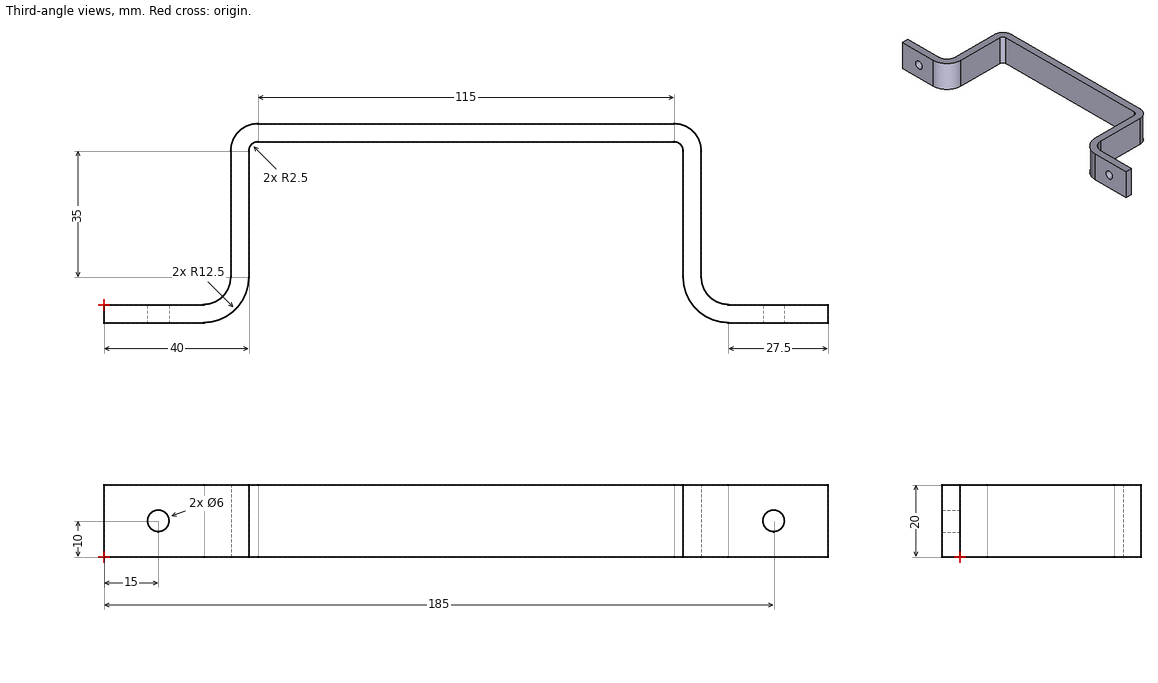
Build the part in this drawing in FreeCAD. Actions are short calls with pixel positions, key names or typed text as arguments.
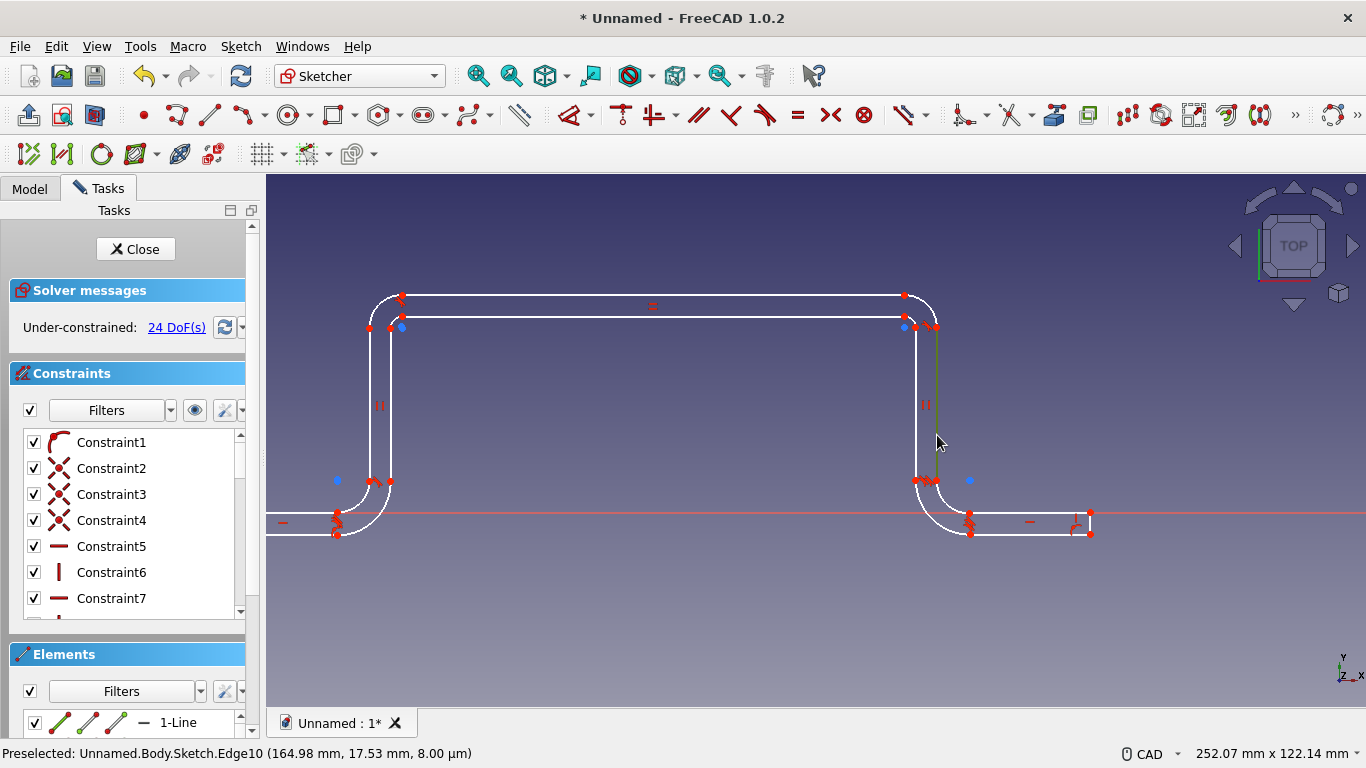
click(933, 313)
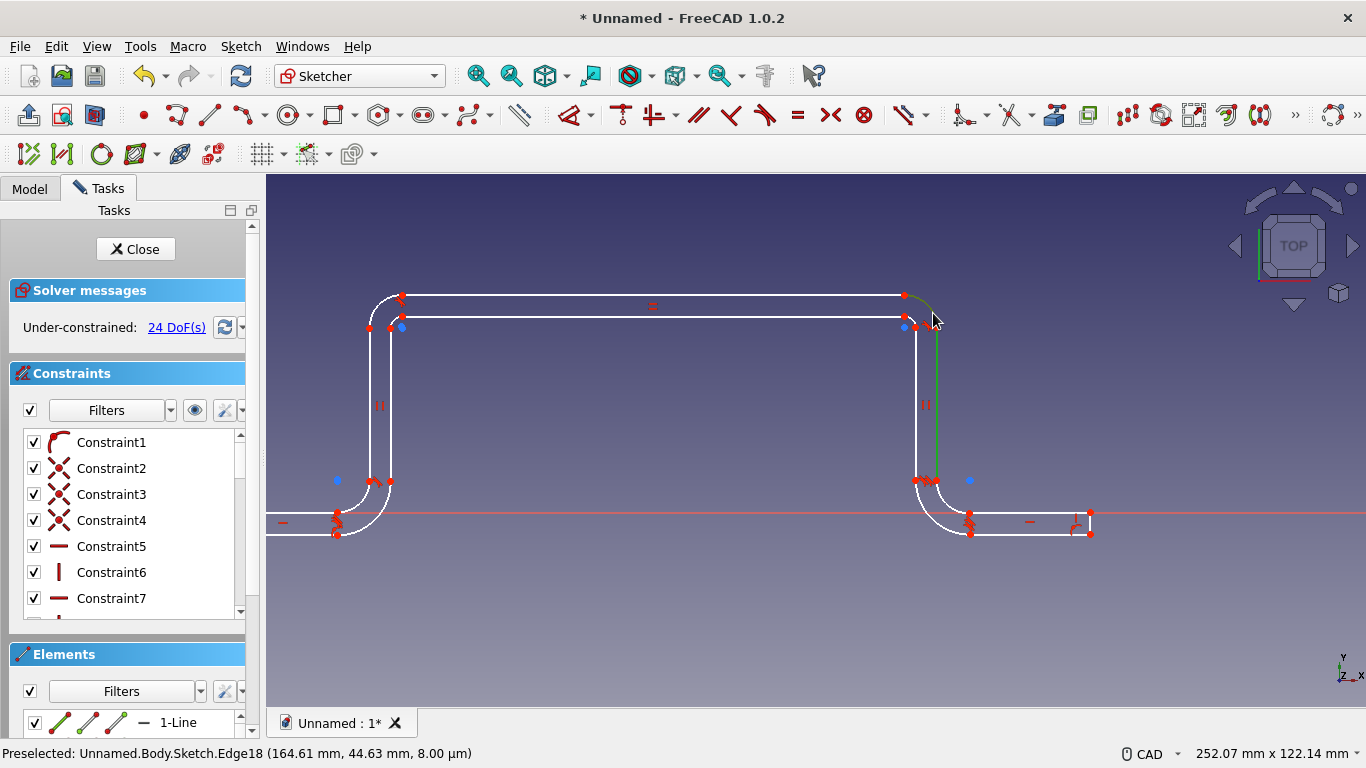
key(t)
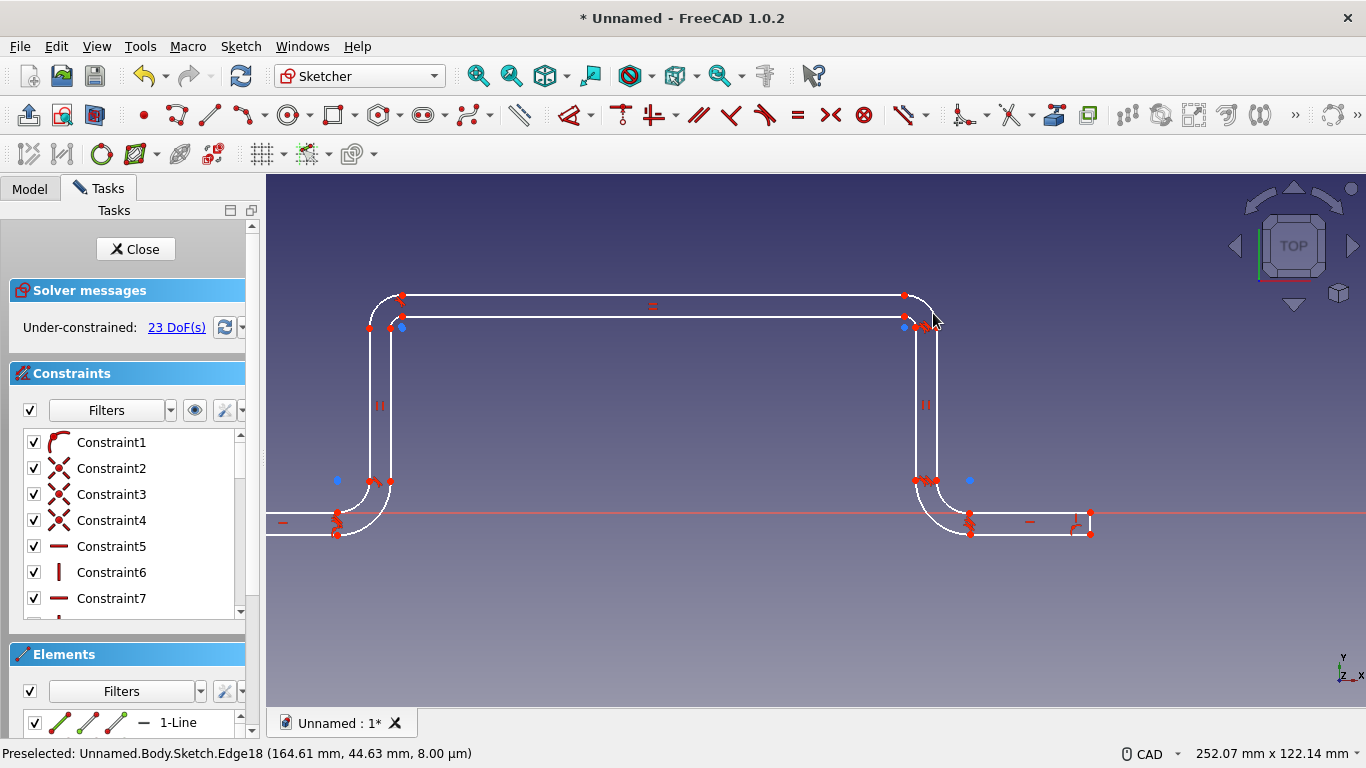
click(754, 295)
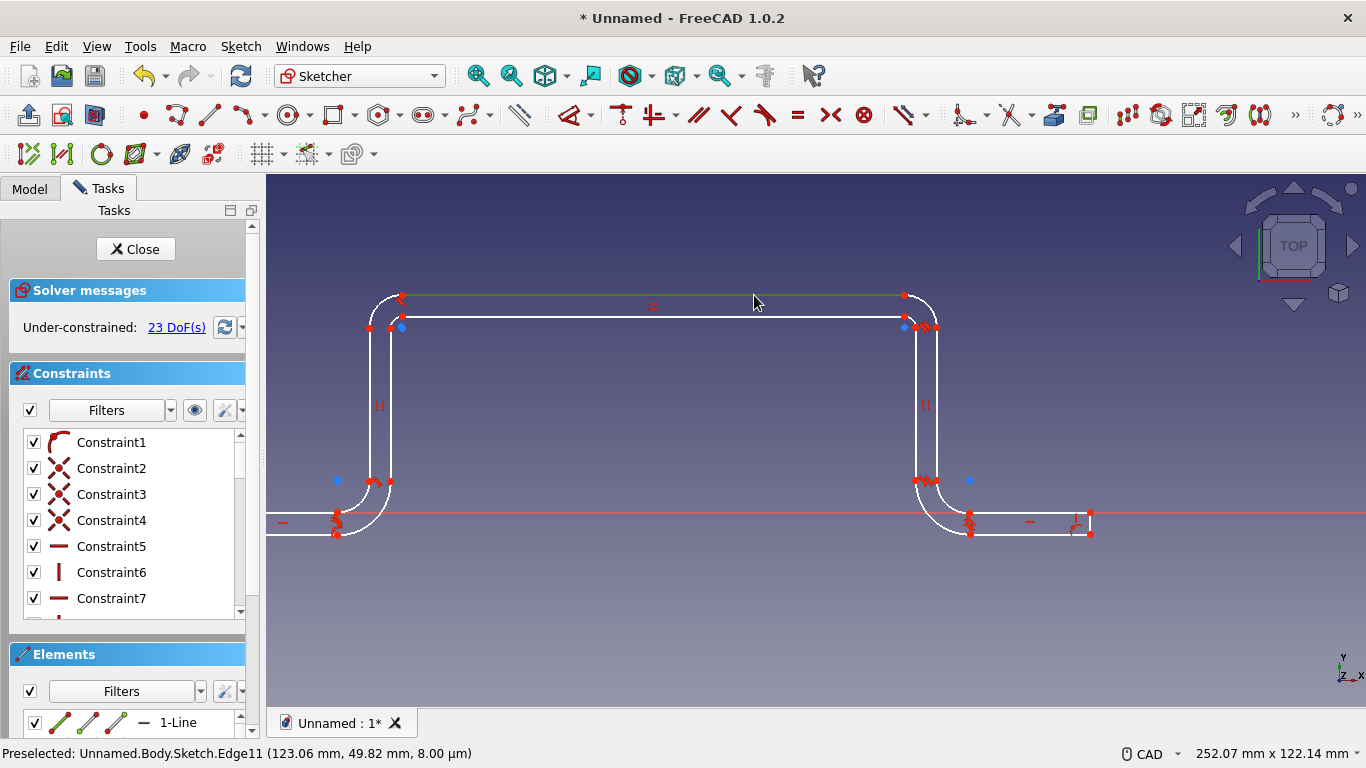
click(933, 313)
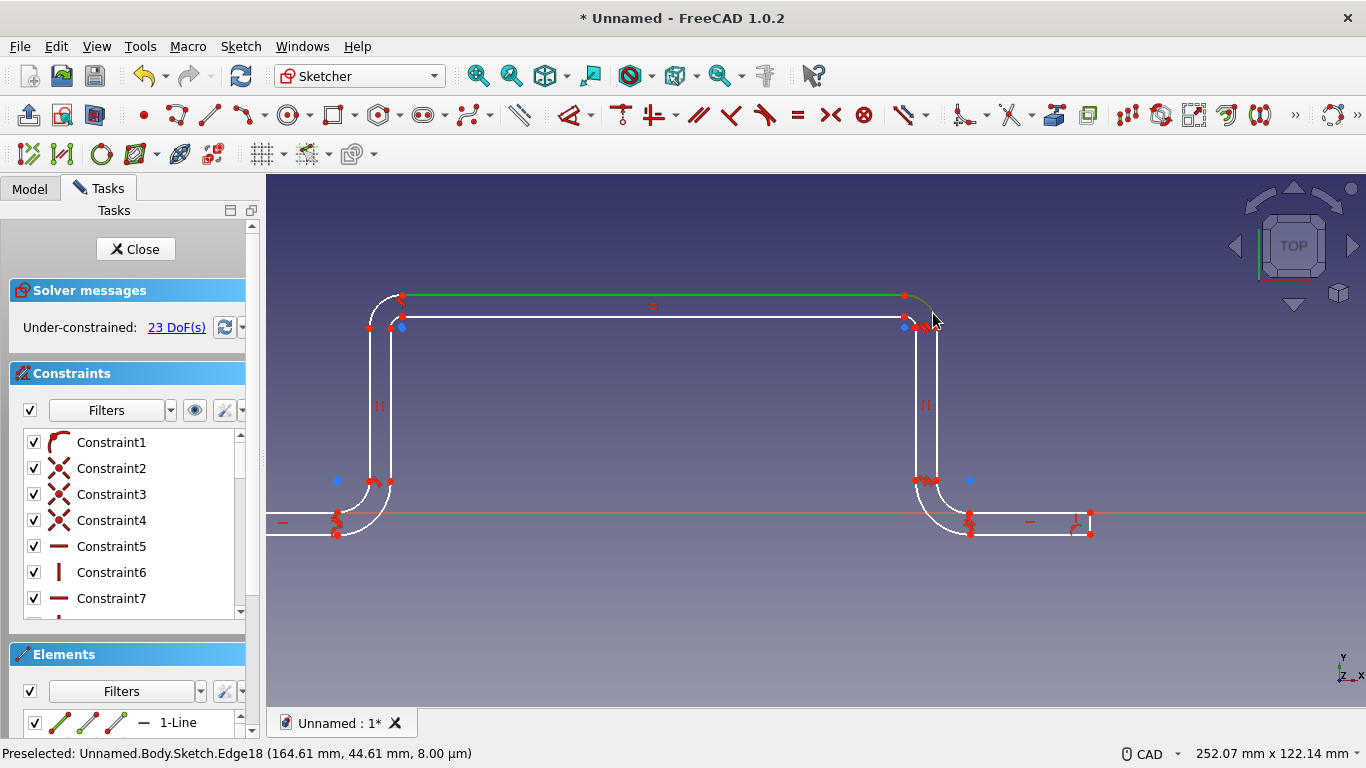
click(765, 116)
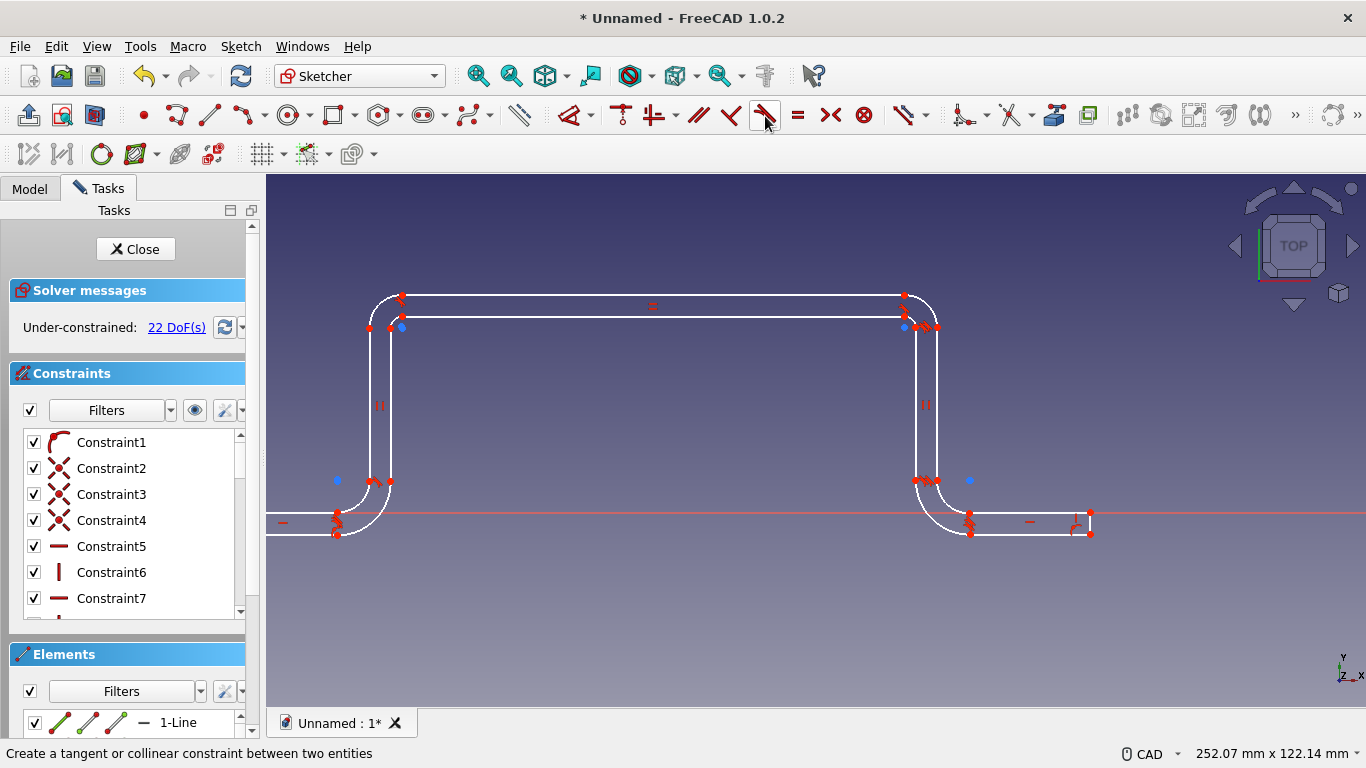
click(754, 295)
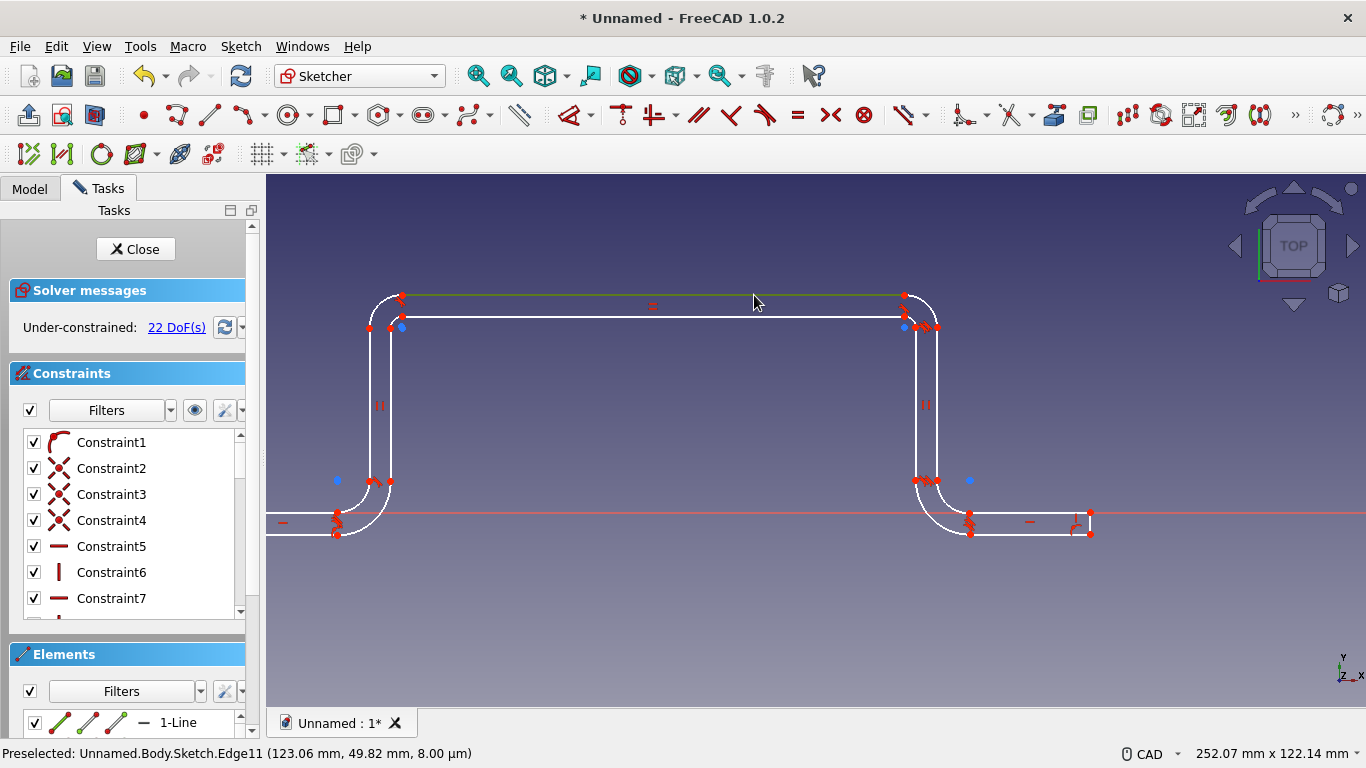
click(387, 299)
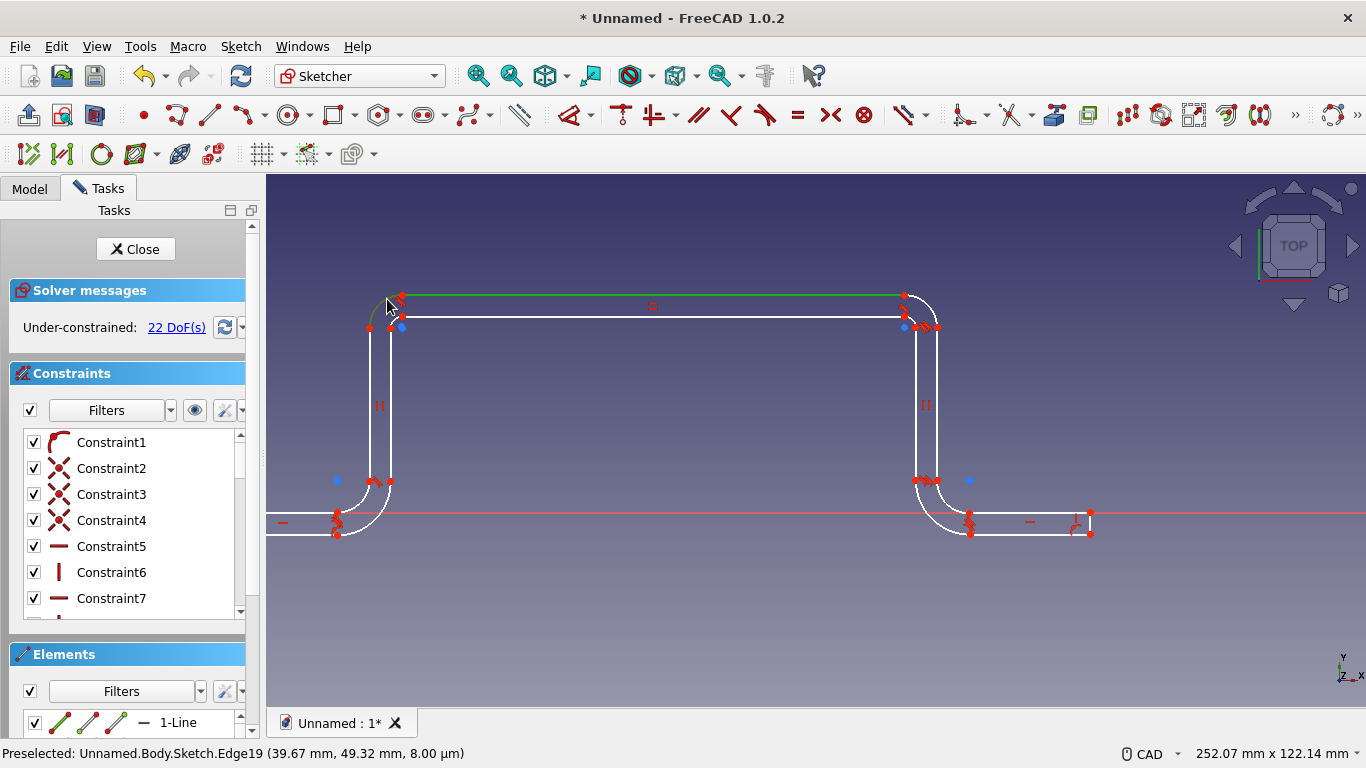
click(765, 116)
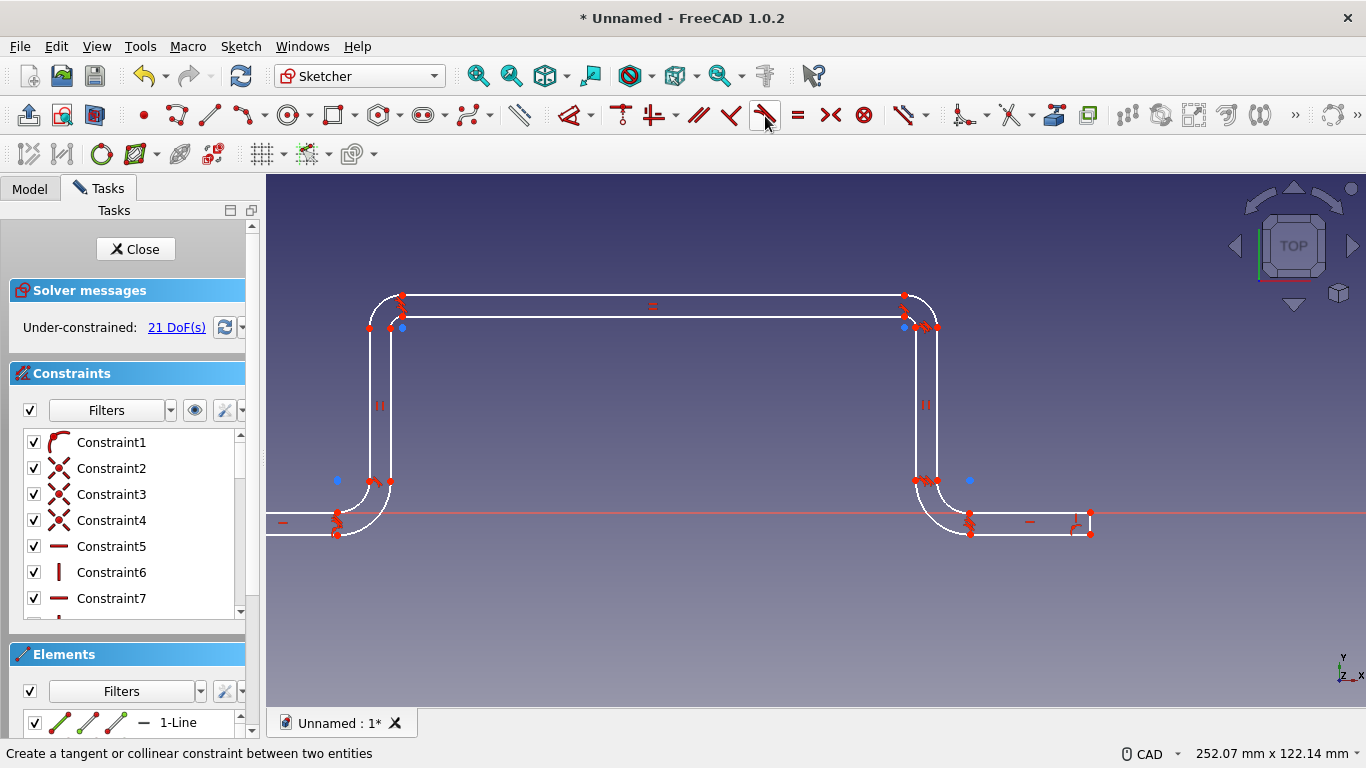
click(370, 374)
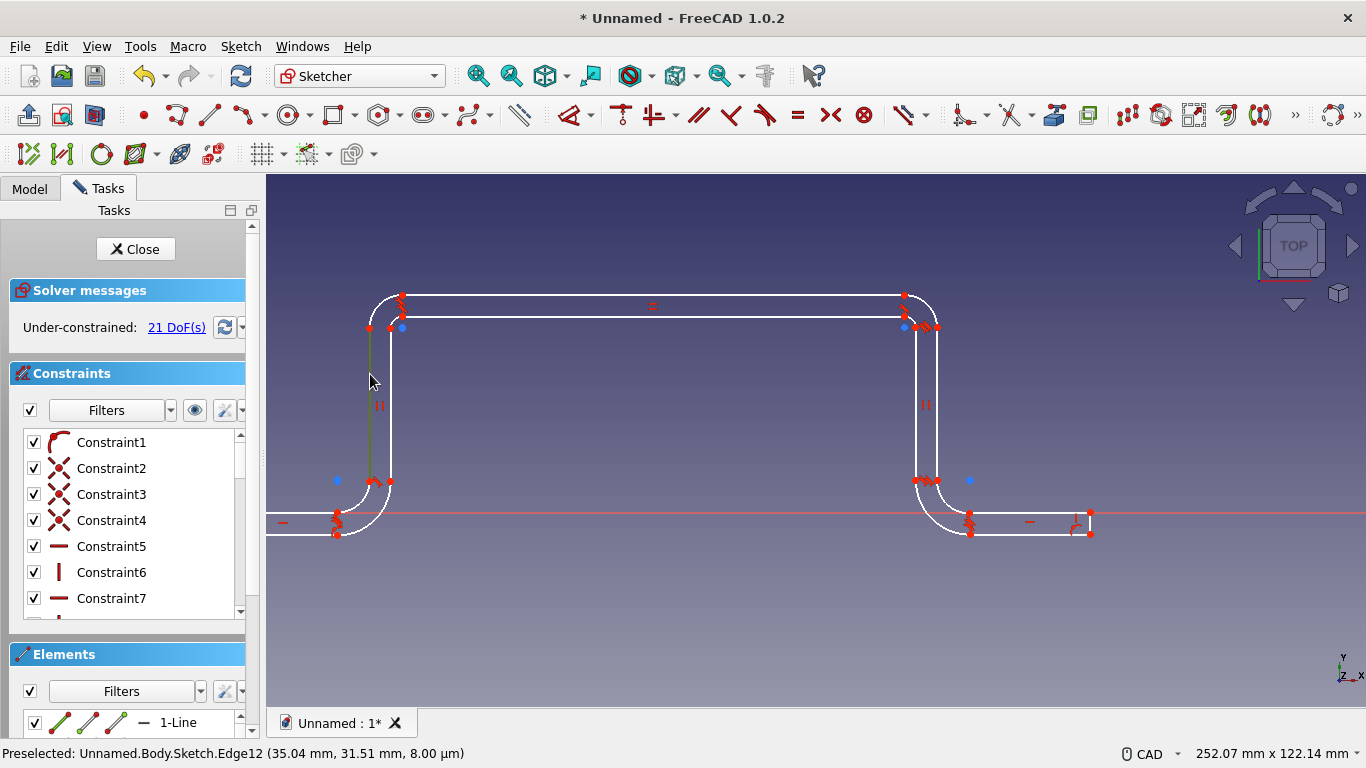
click(387, 299)